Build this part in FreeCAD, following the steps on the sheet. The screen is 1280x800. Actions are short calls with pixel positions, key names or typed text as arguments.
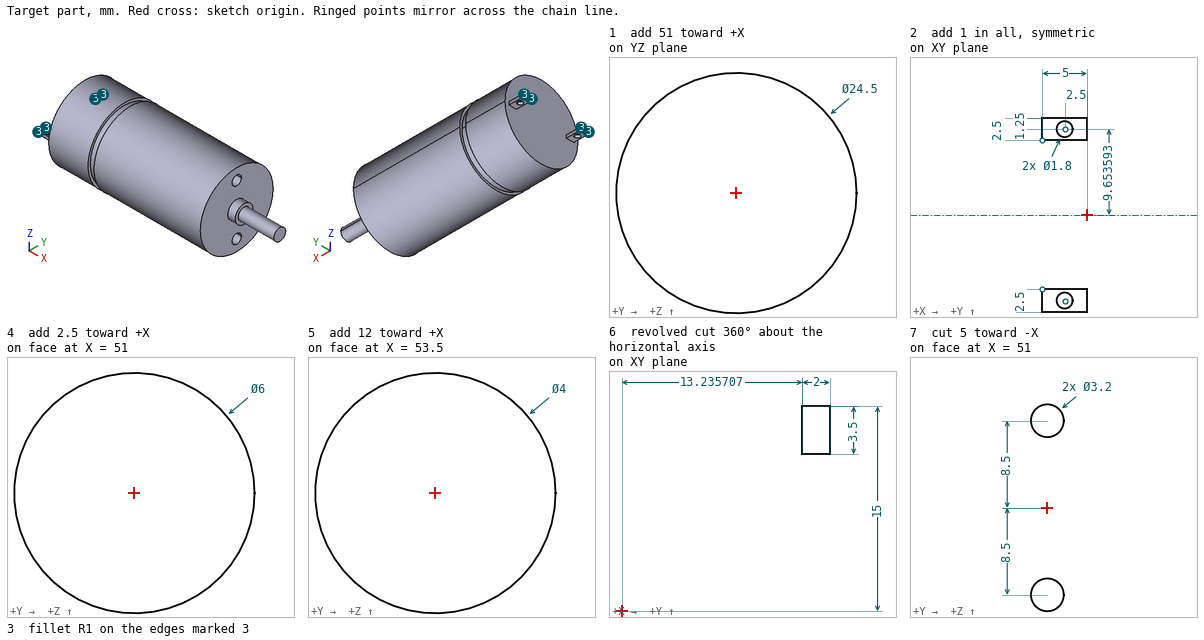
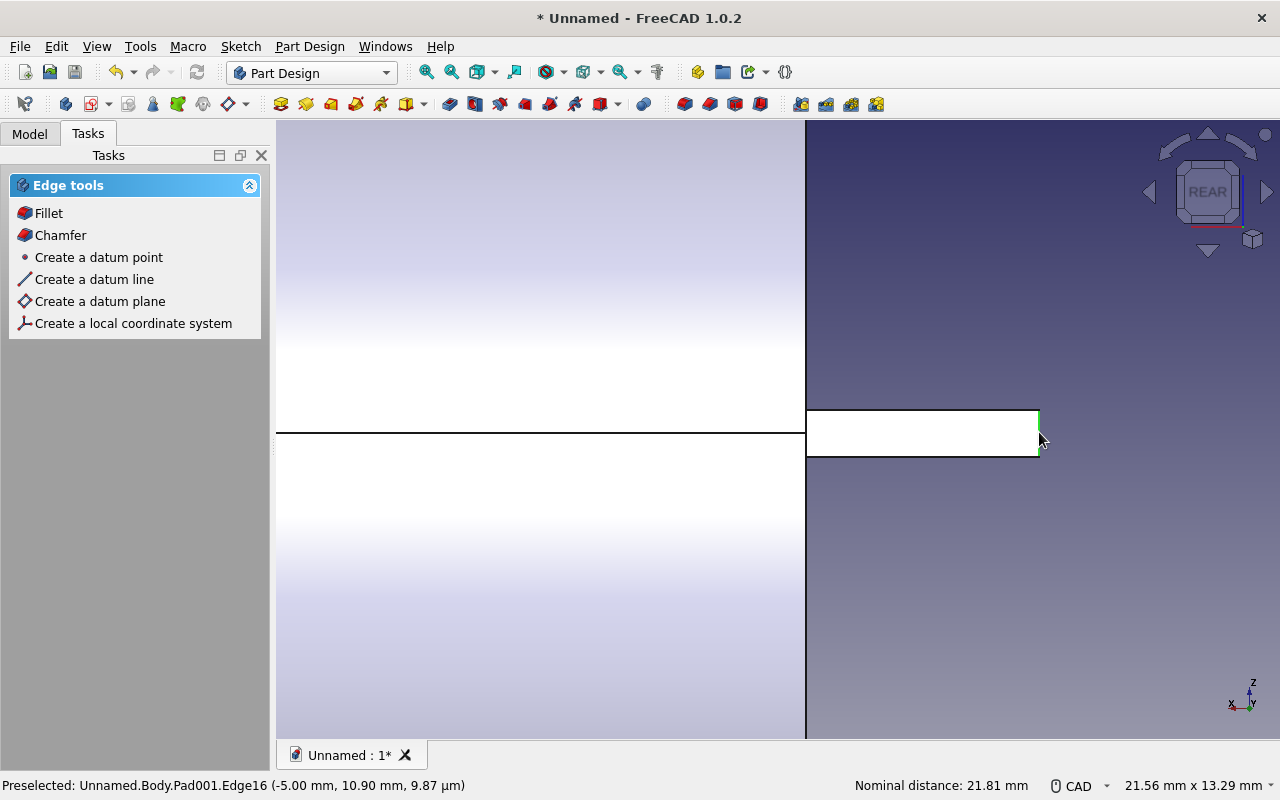
click(427, 72)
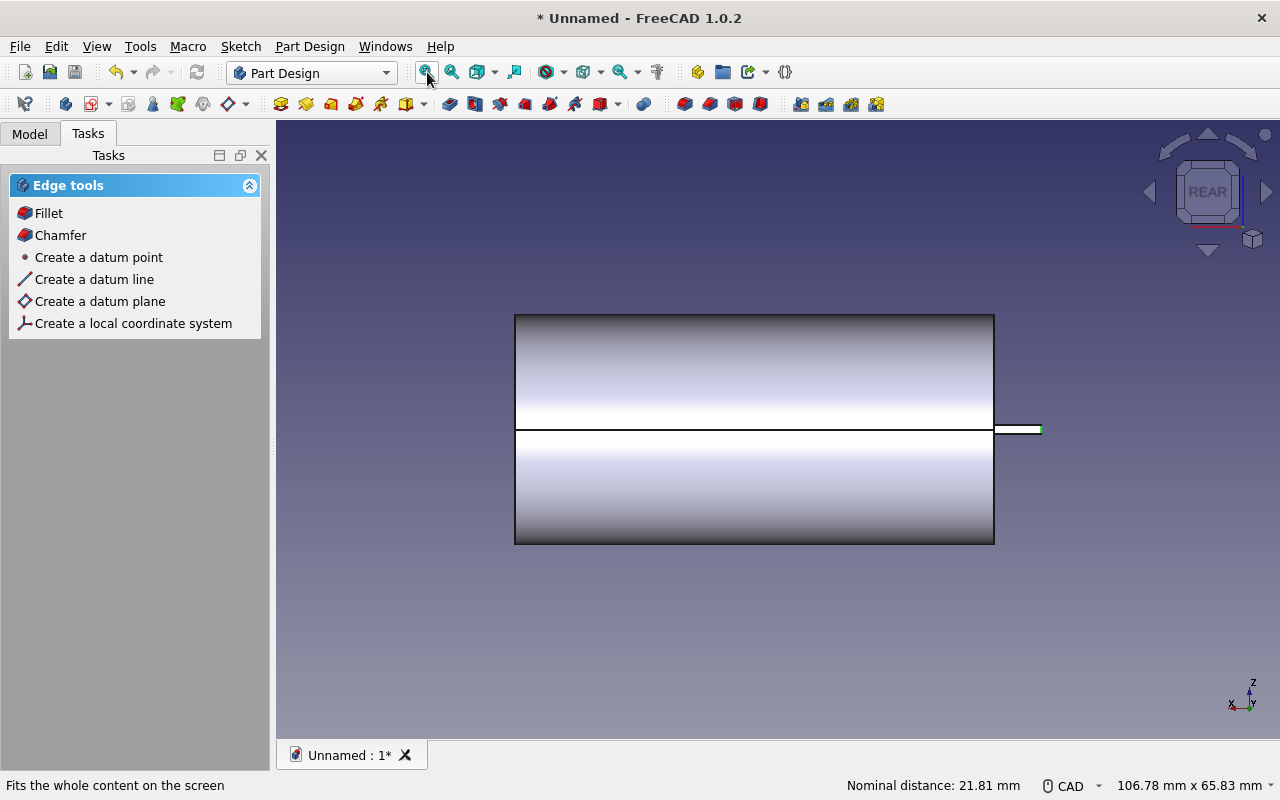
key(6)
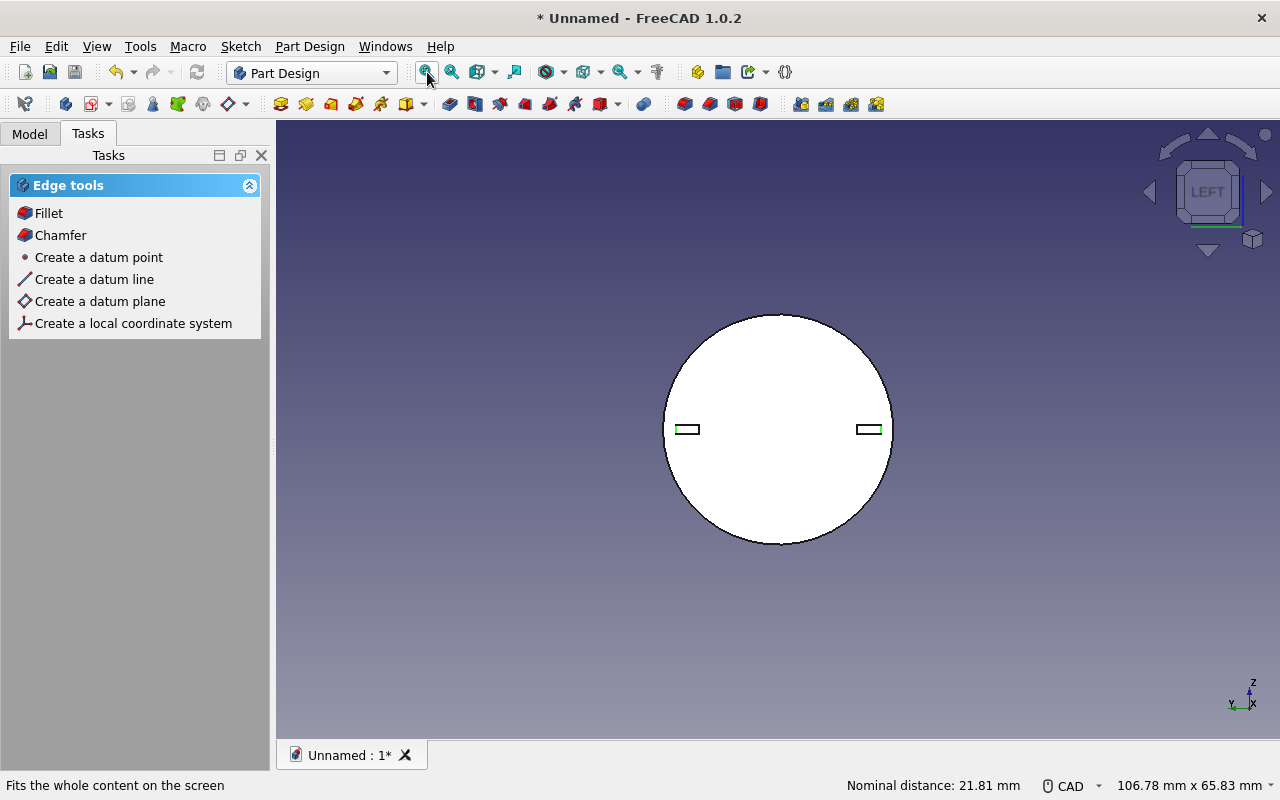
click(427, 72)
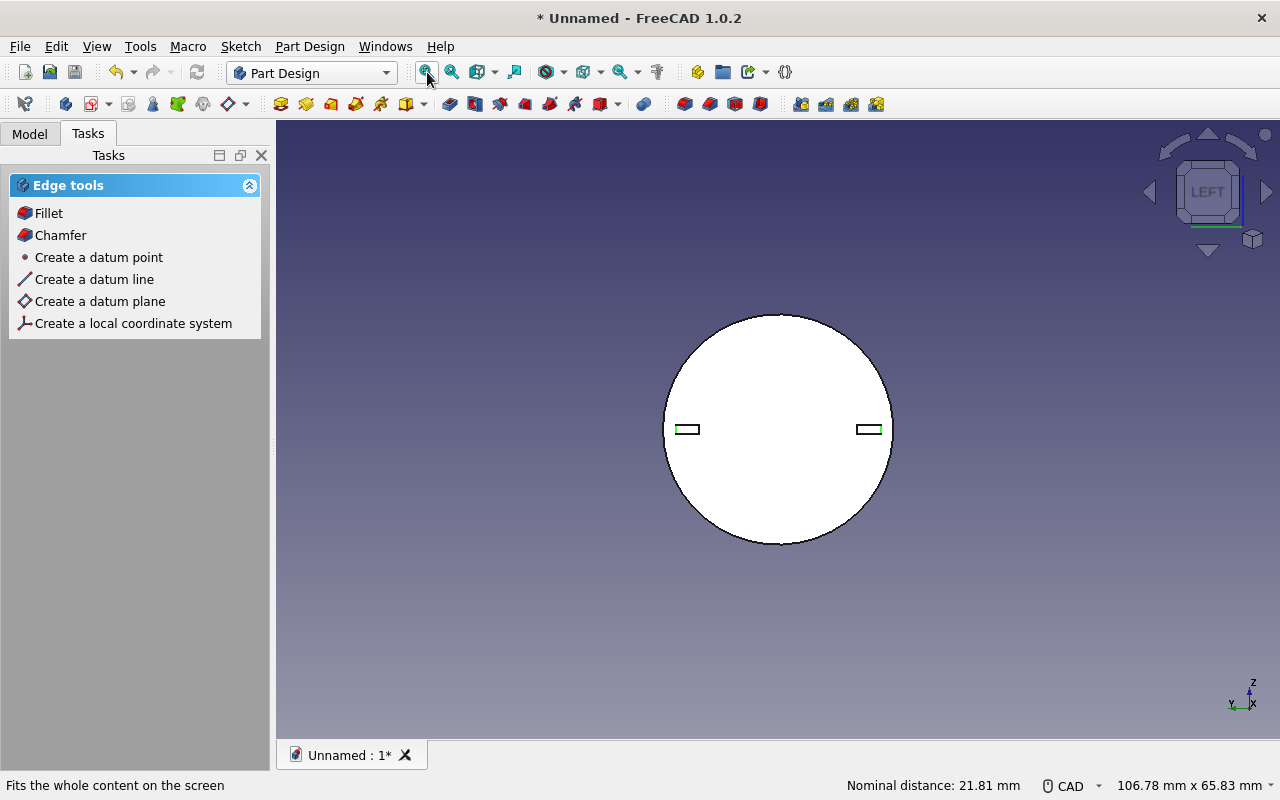
scroll(699, 428, up, 8)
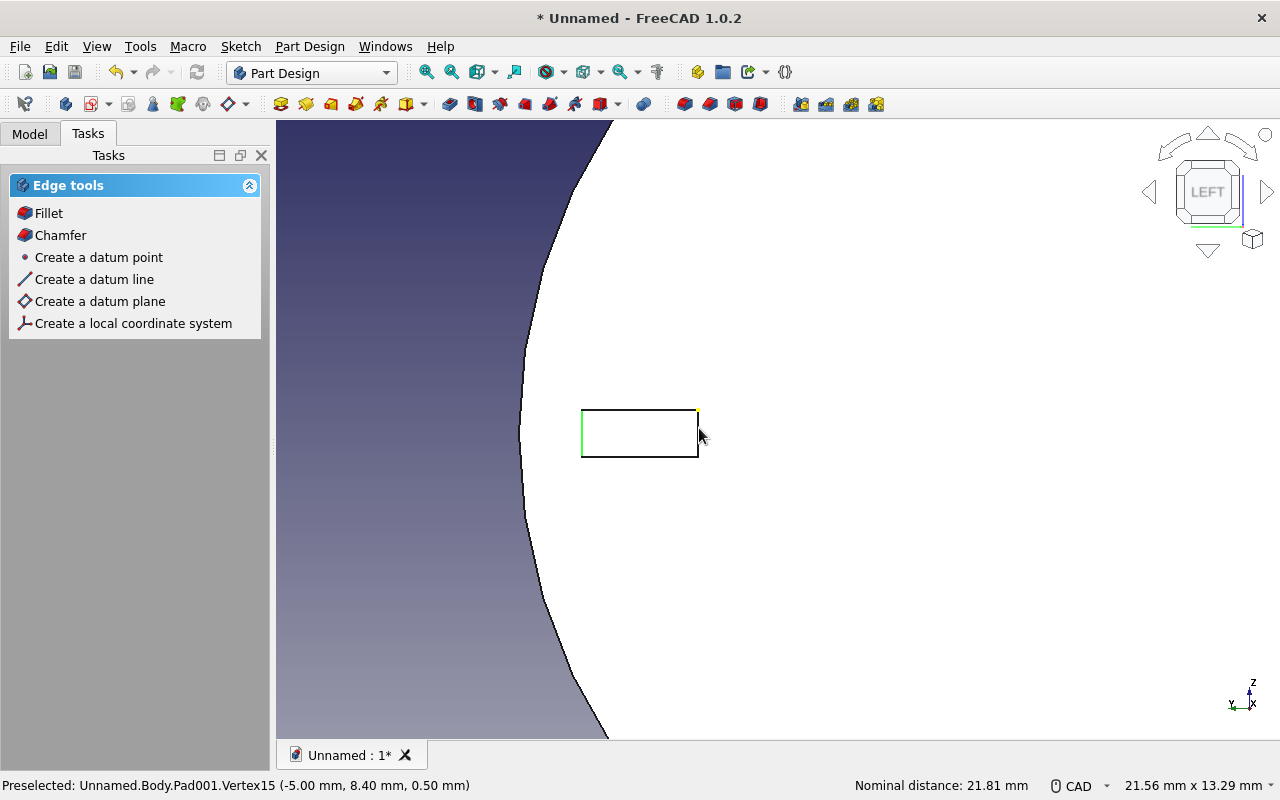
click(698, 432, ctrl)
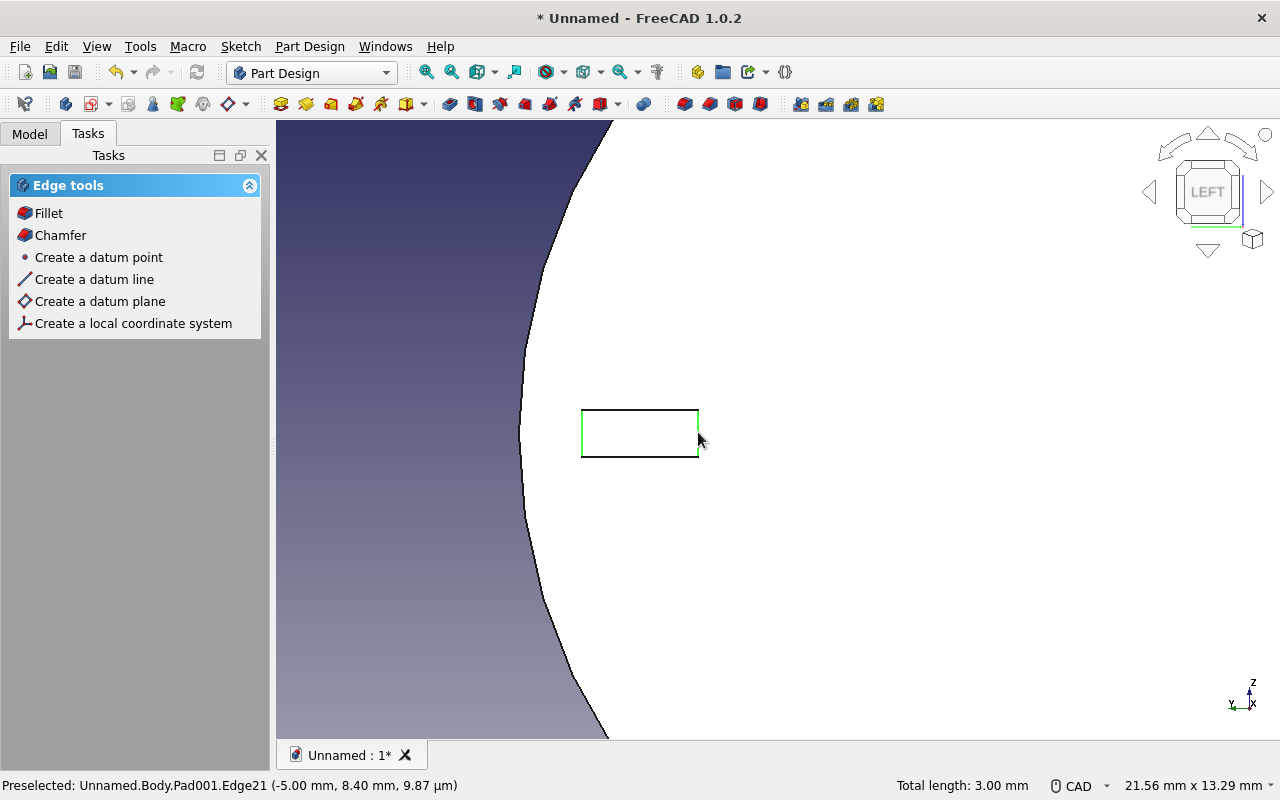
click(427, 72)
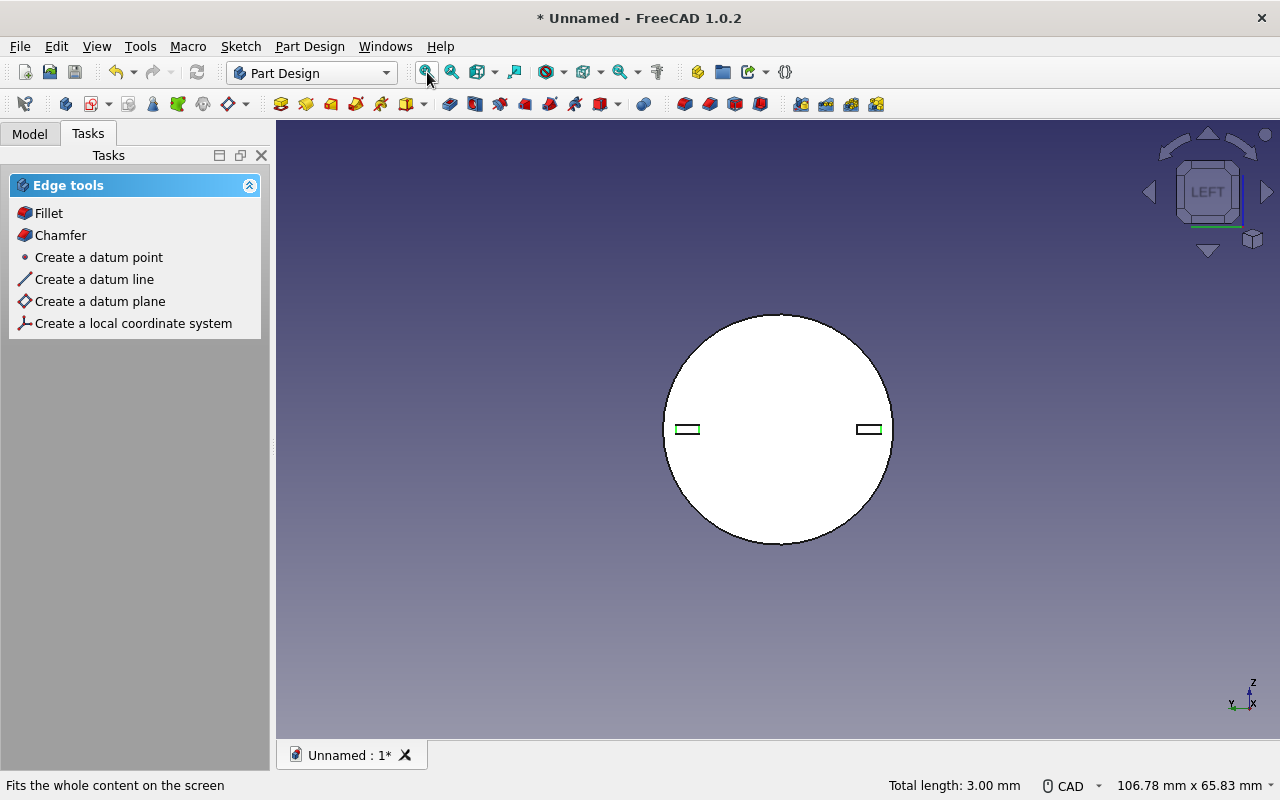
key(v)
key(3)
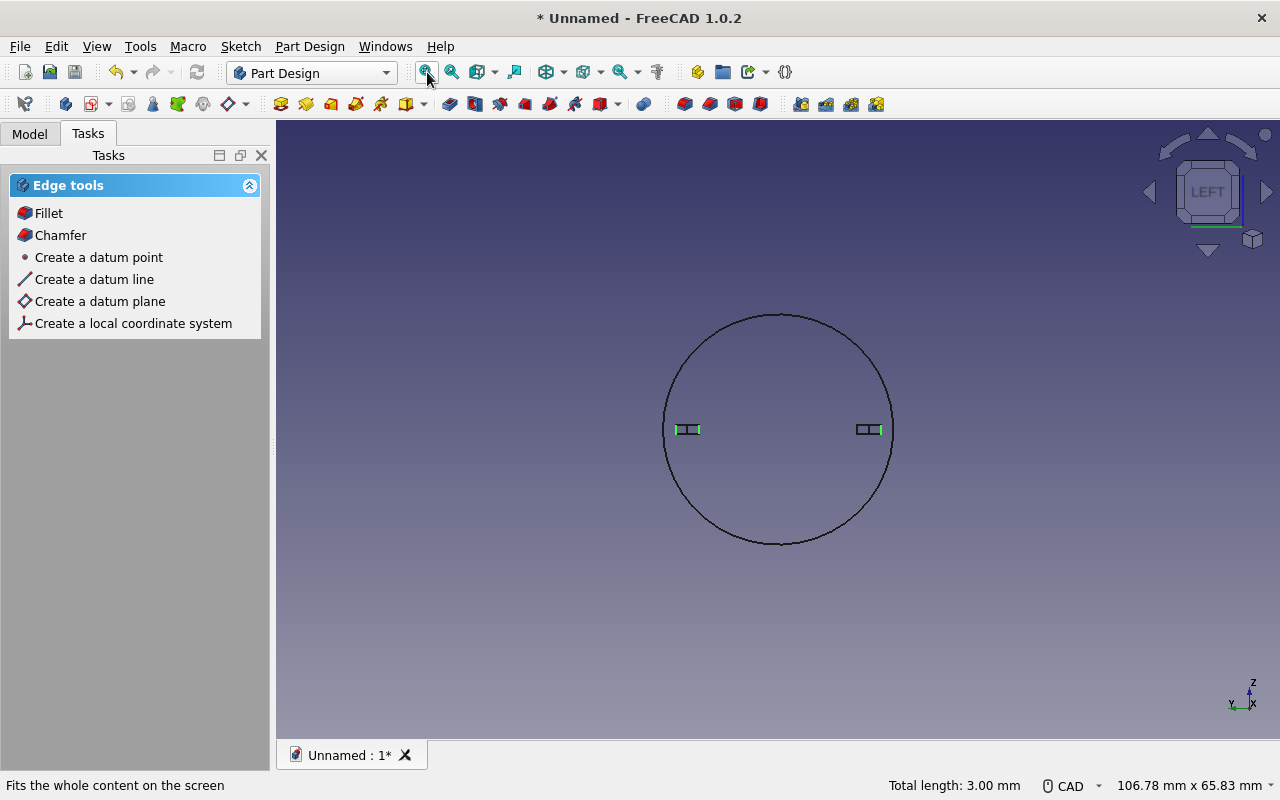
key(0)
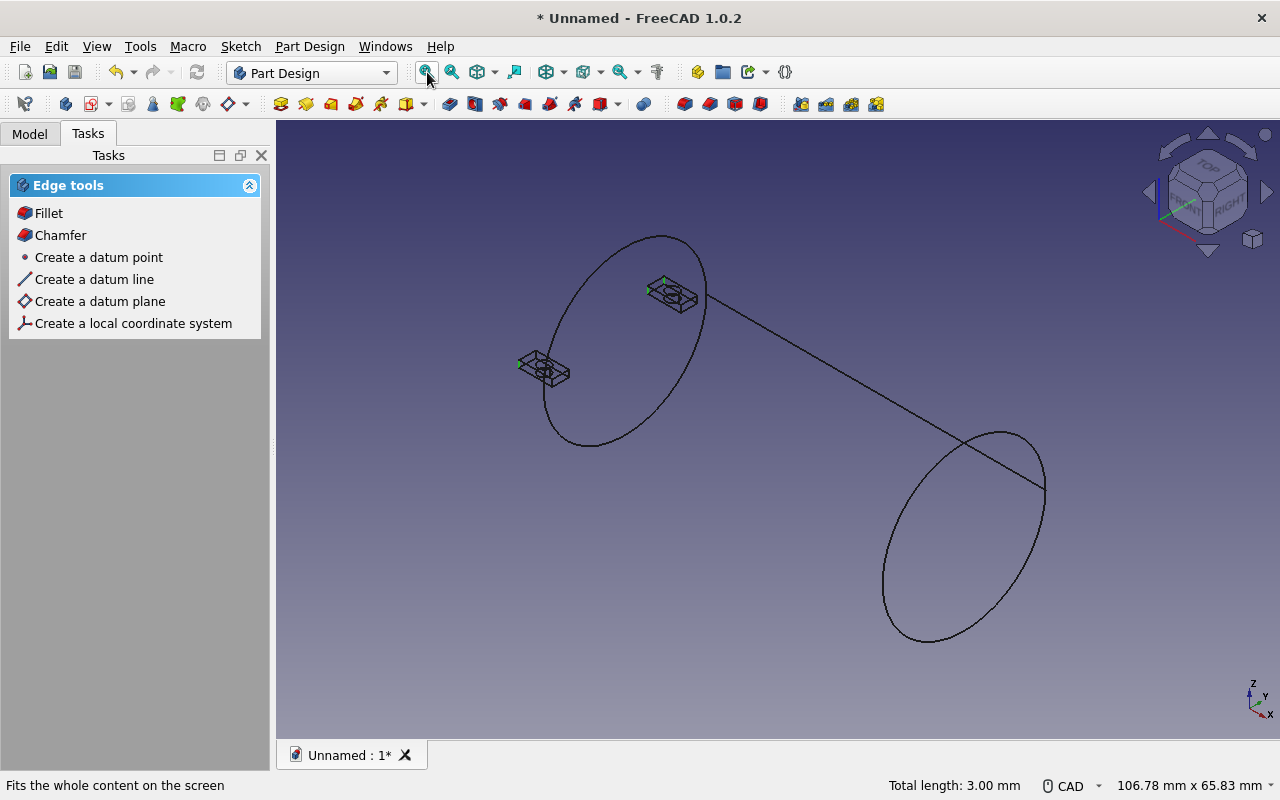
scroll(536, 353, up, 8)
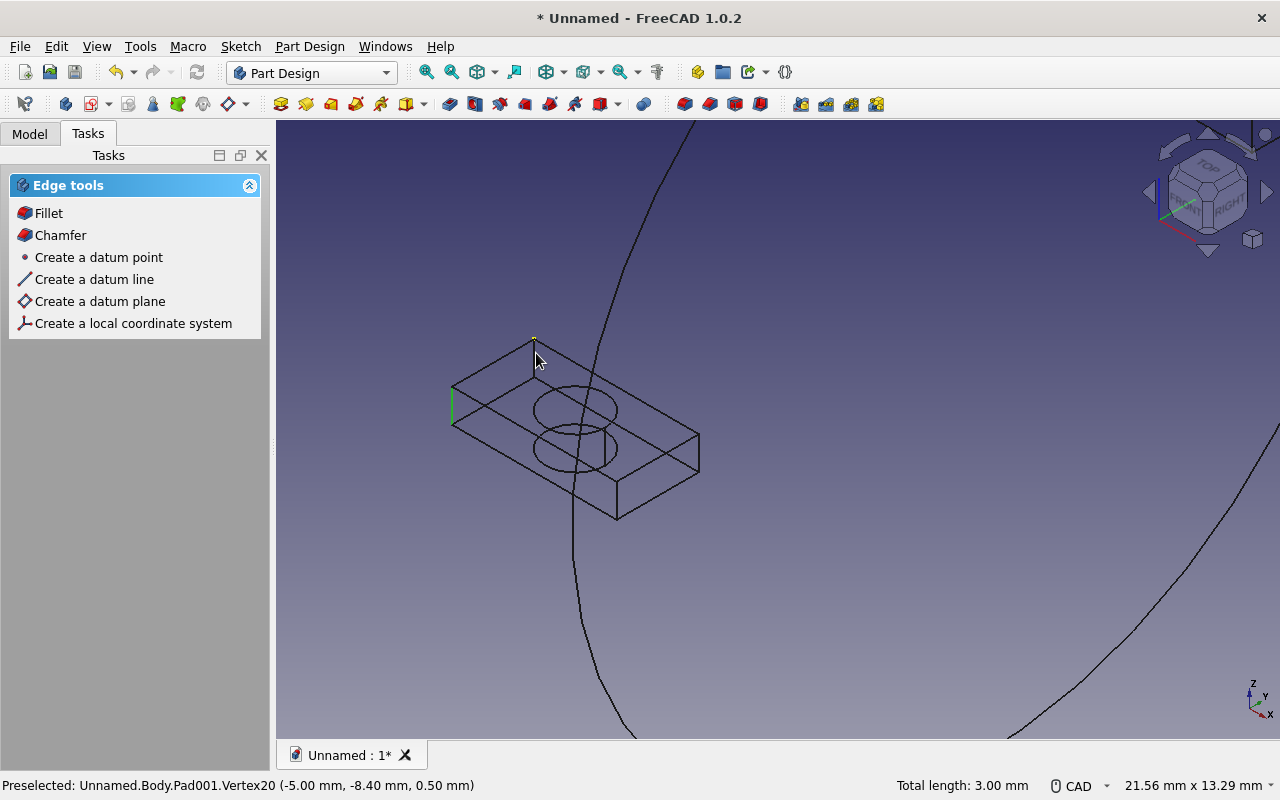
click(534, 357, ctrl)